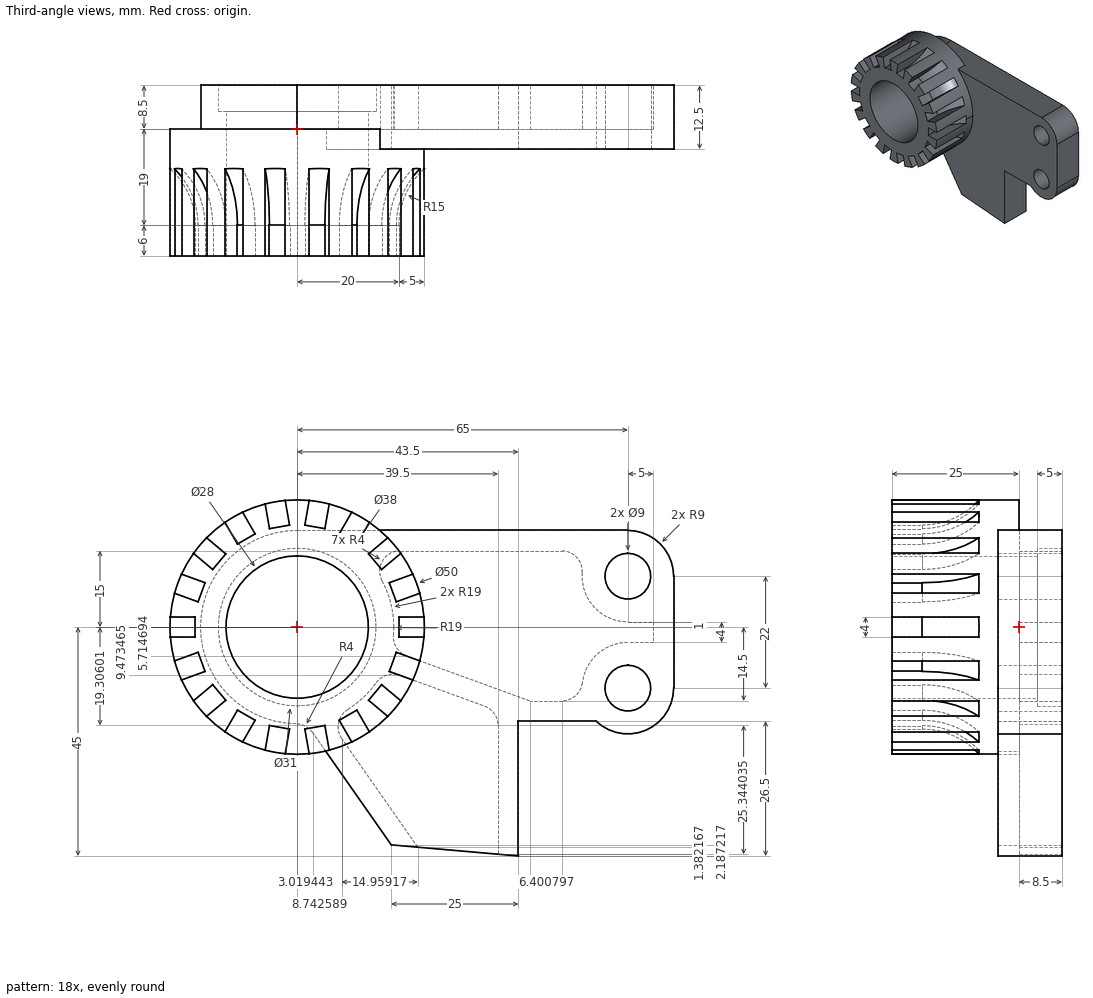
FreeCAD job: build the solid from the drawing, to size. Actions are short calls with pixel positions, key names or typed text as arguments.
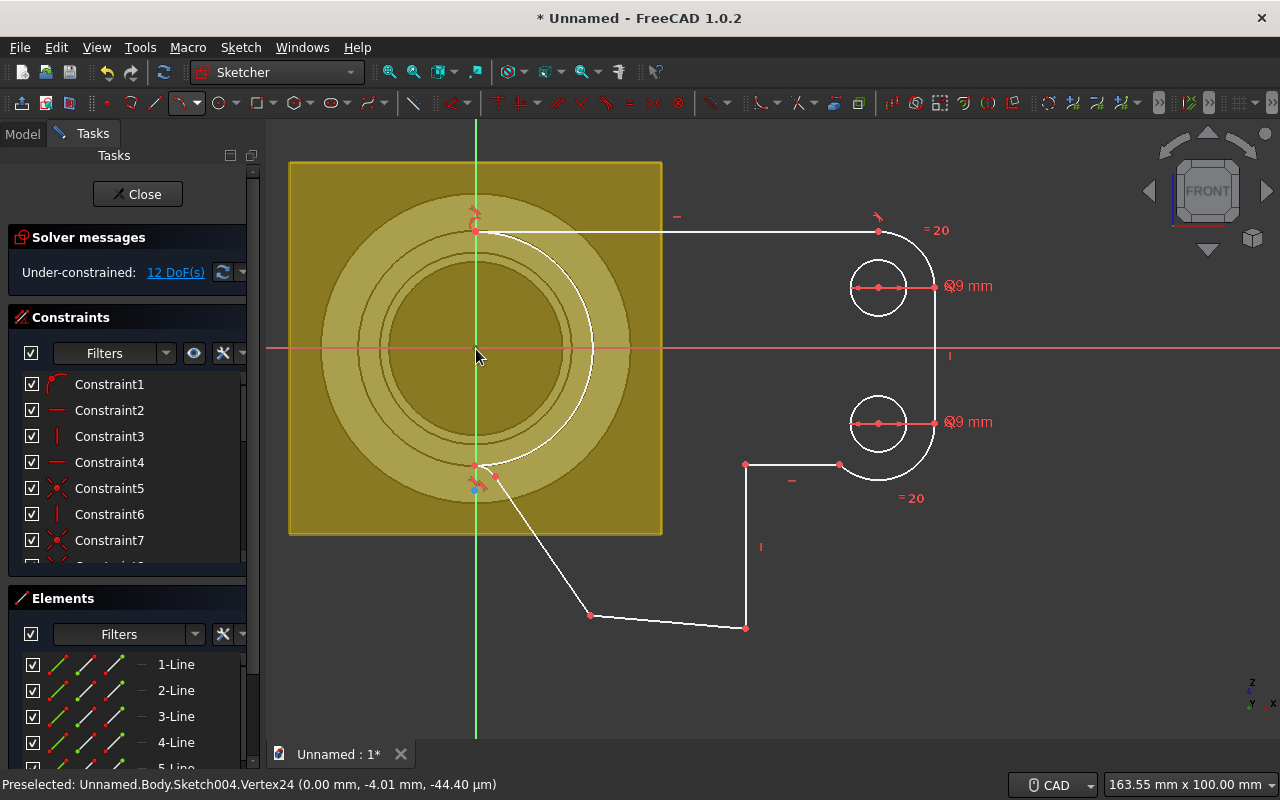
click(353, 348)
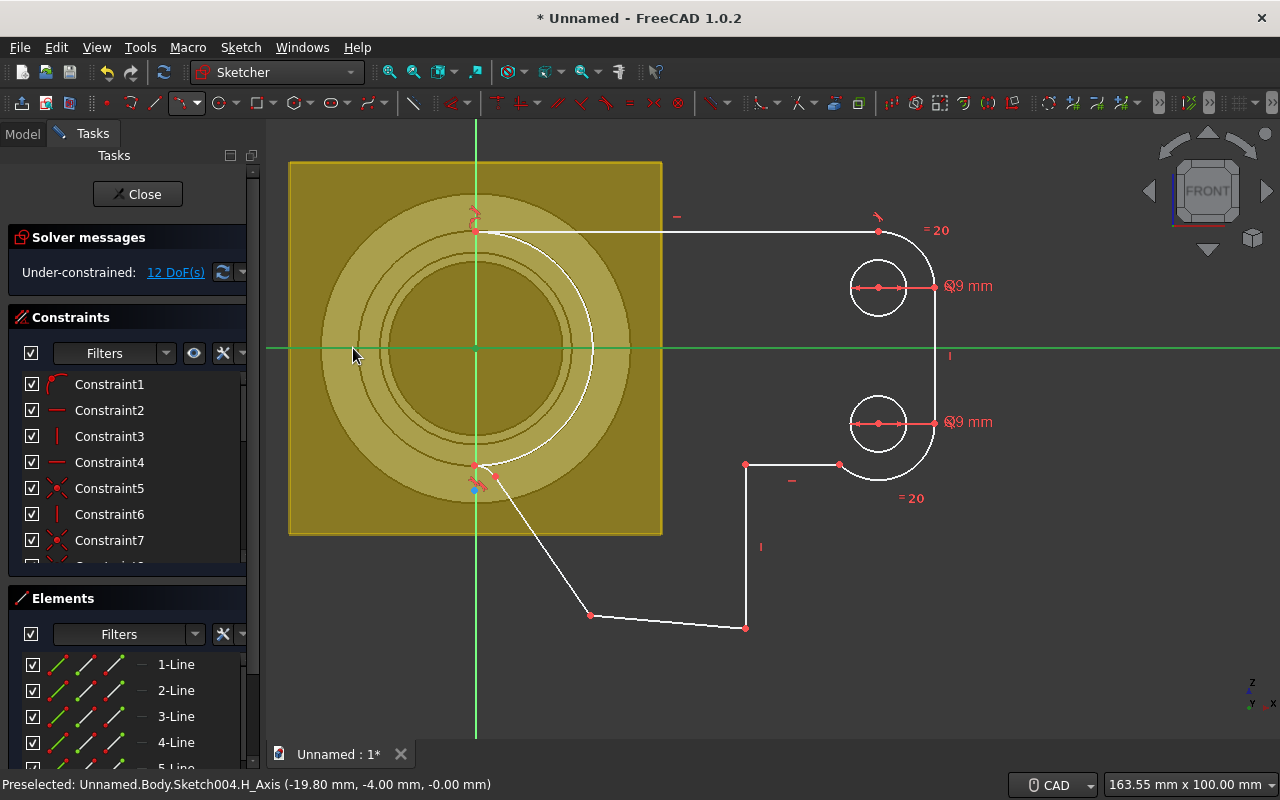
click(498, 104)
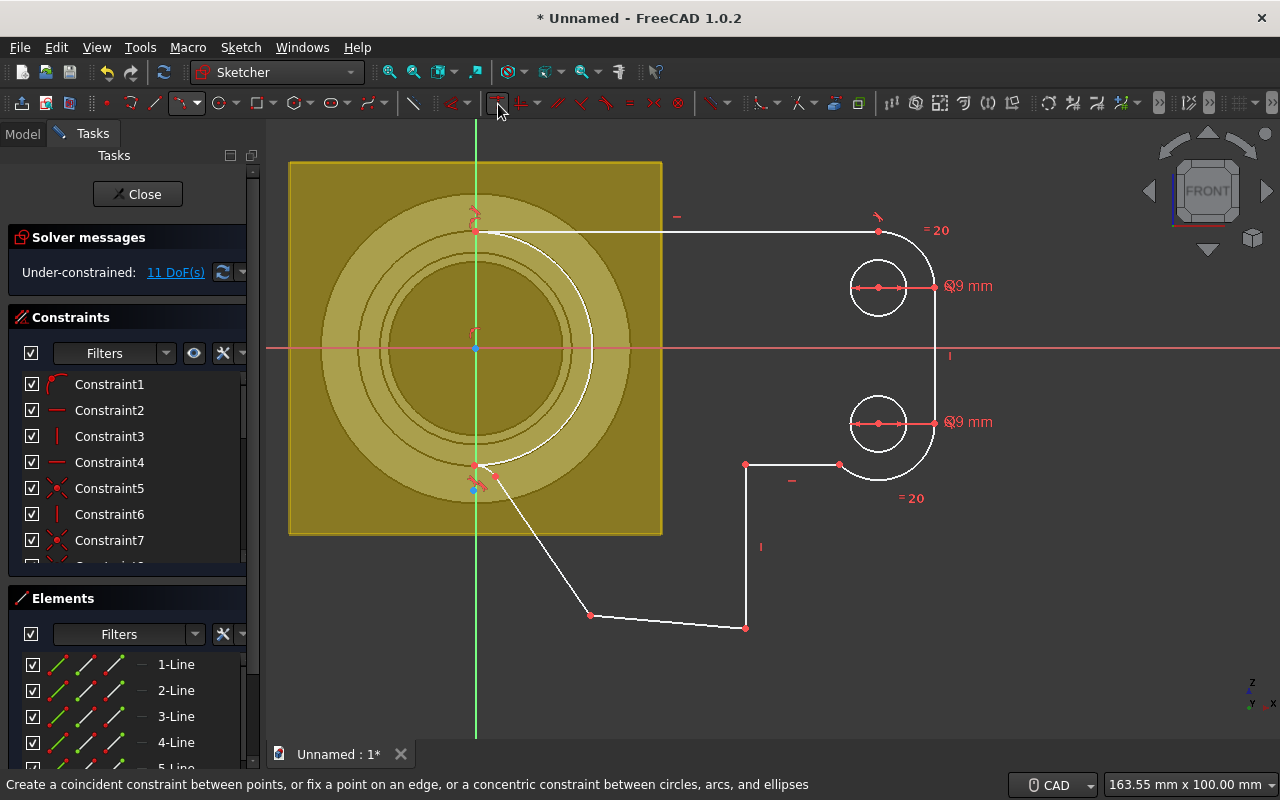
click(452, 104)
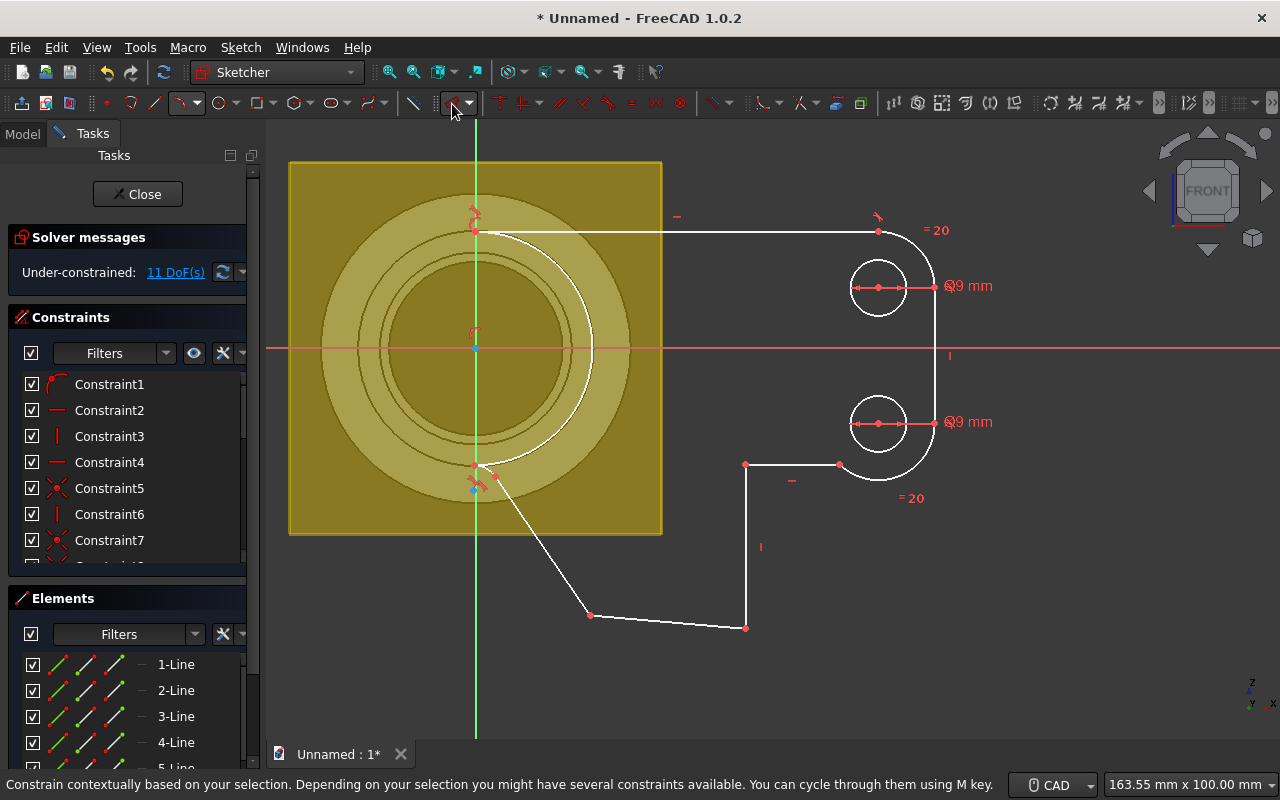
click(928, 262)
click(956, 247)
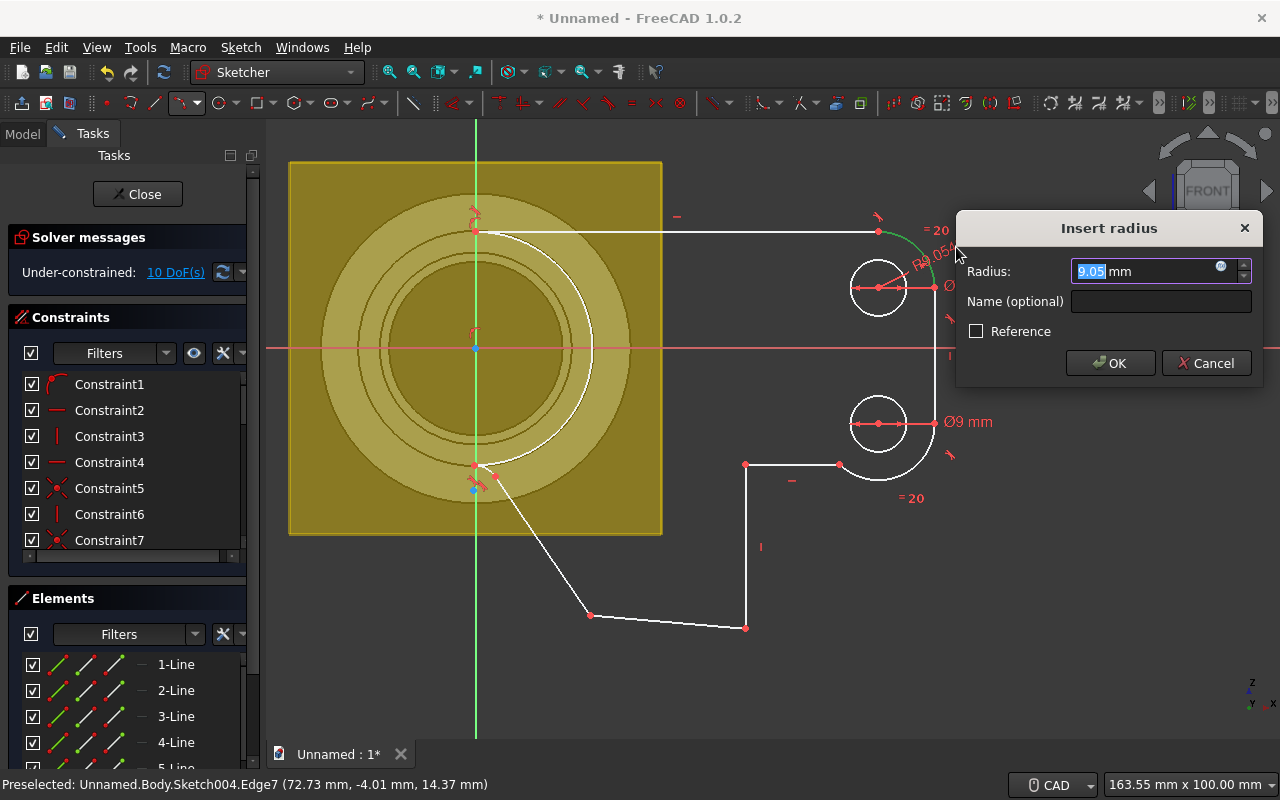
text(9)
key(Return)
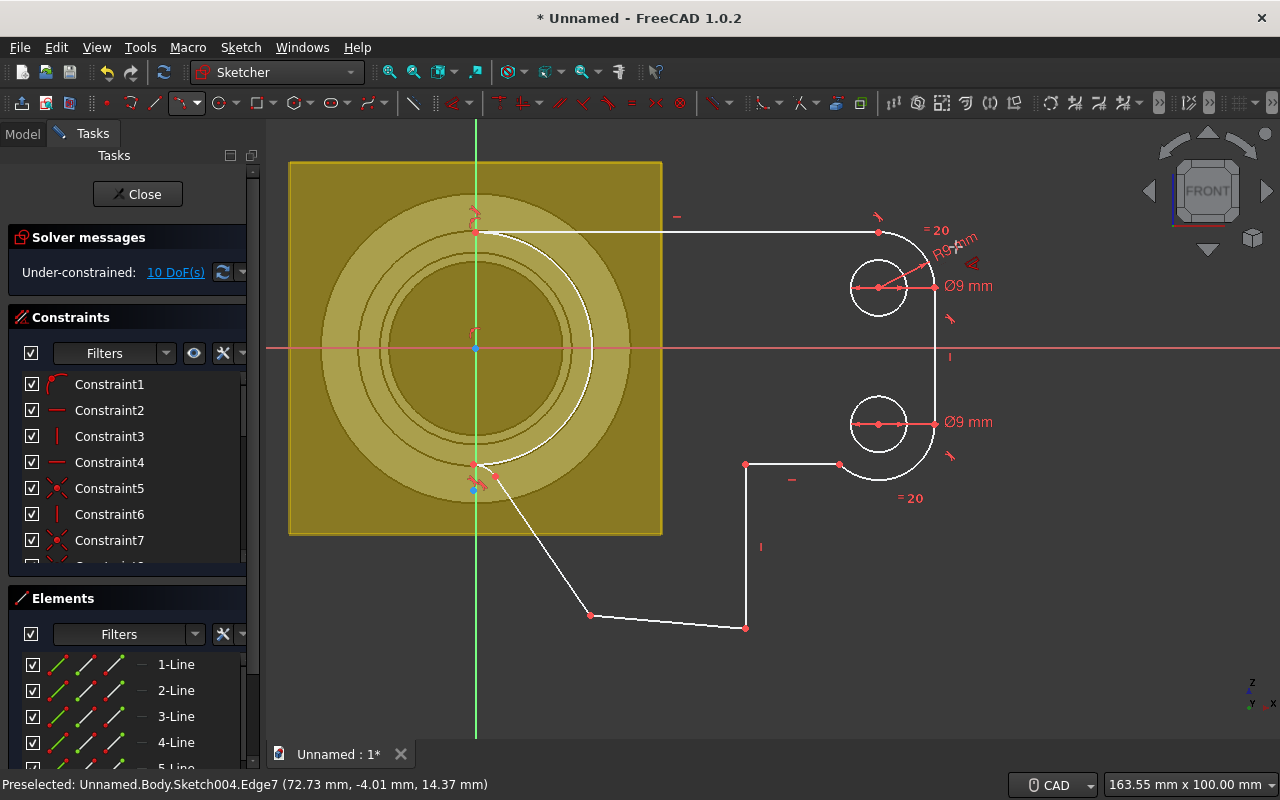
scroll(490, 471, up, 4)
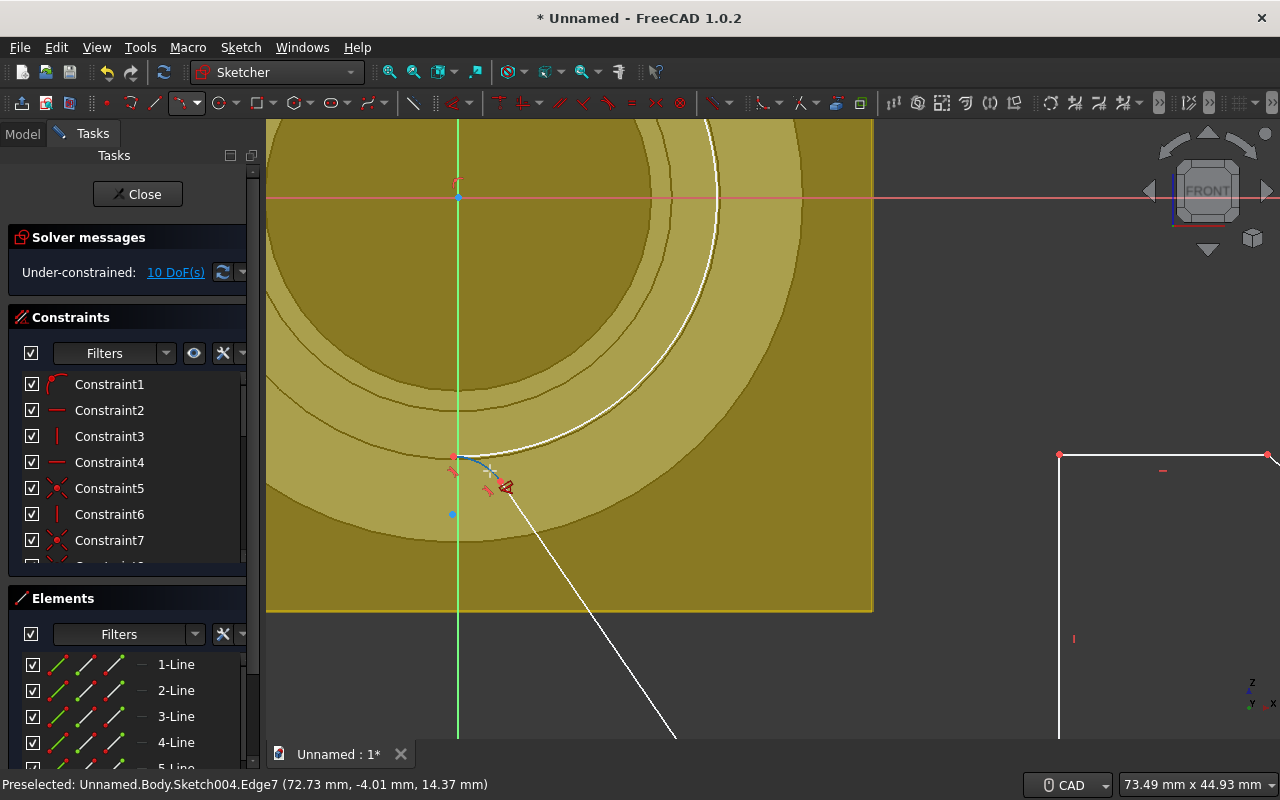
click(490, 470)
click(537, 481)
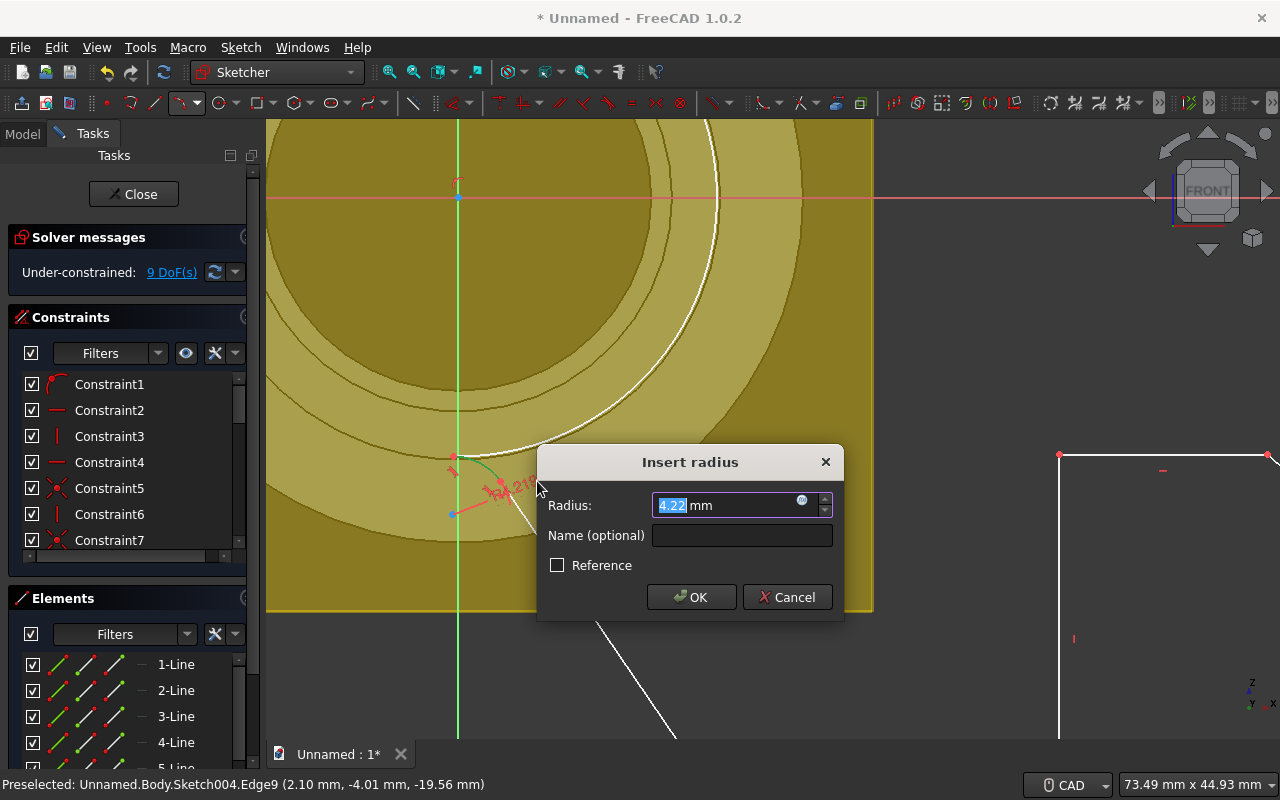
text(4)
key(Return)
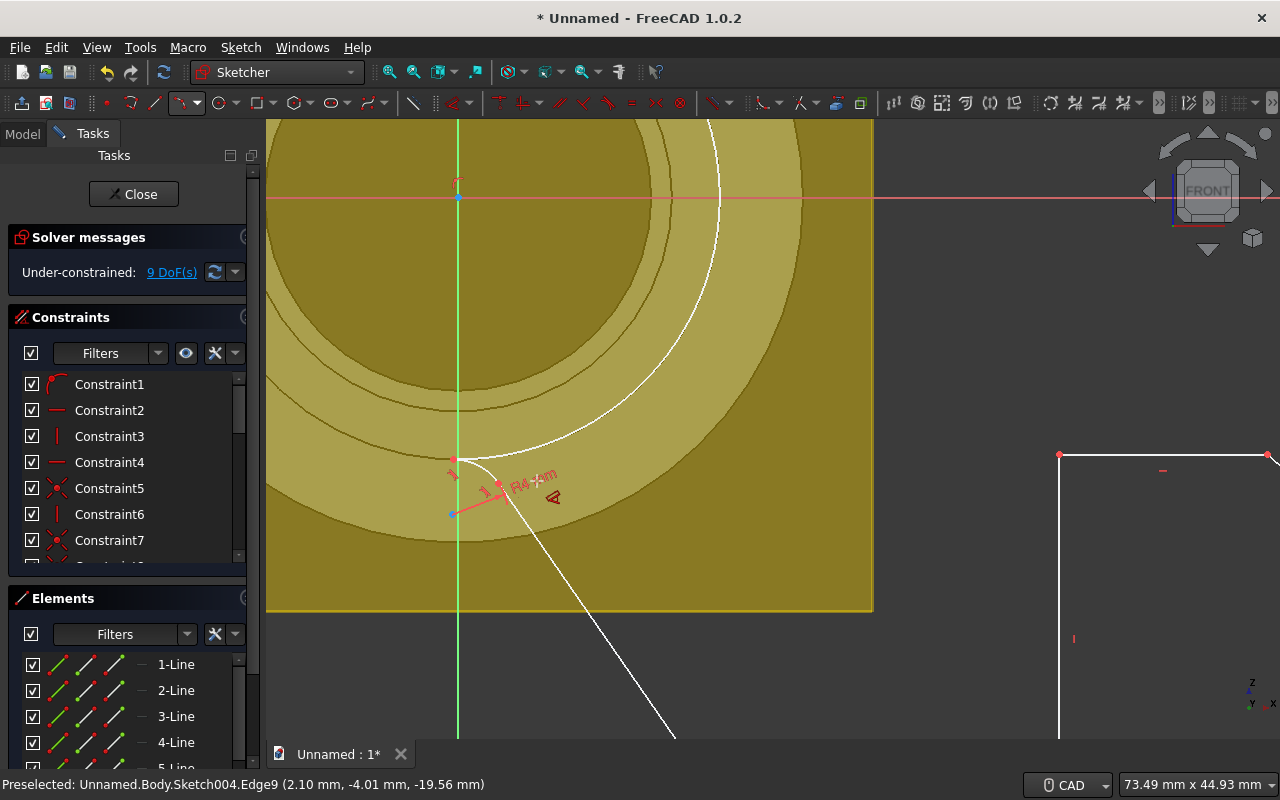
click(668, 354)
click(694, 373)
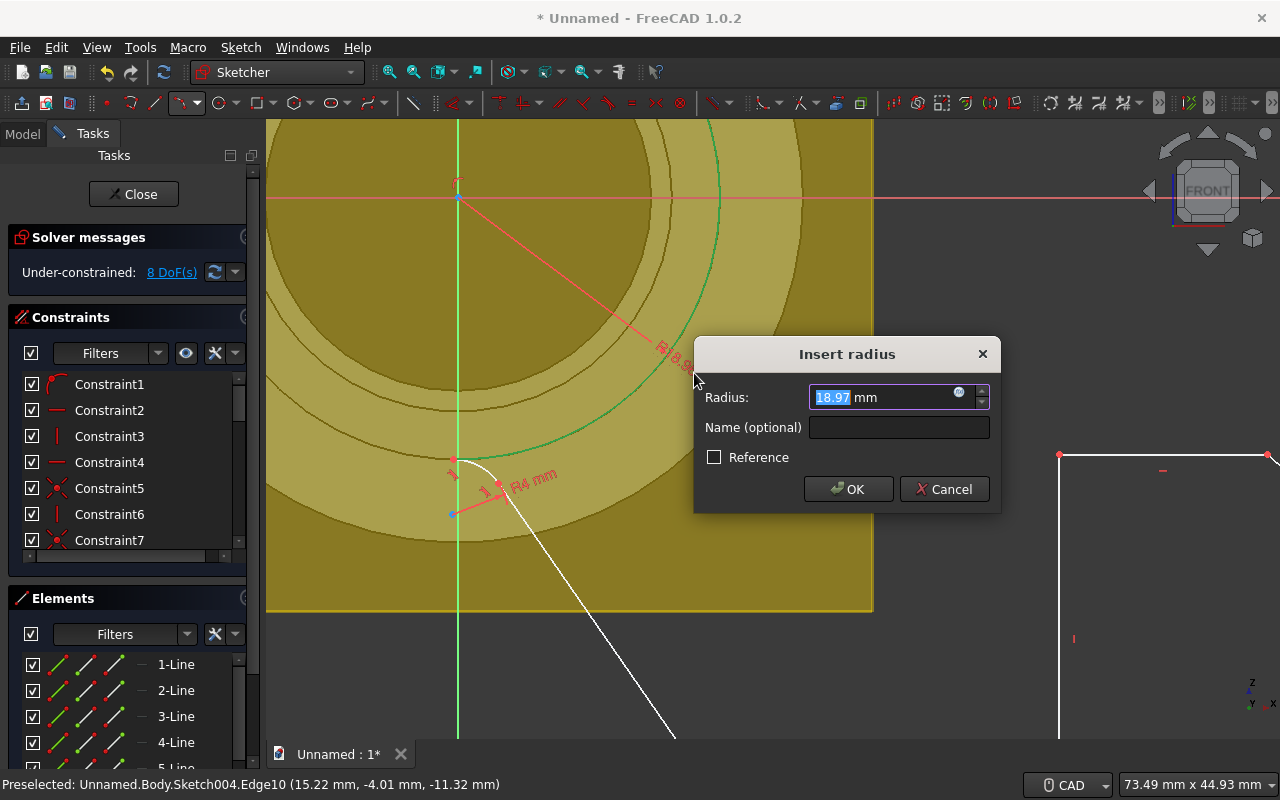
text(19)
key(Return)